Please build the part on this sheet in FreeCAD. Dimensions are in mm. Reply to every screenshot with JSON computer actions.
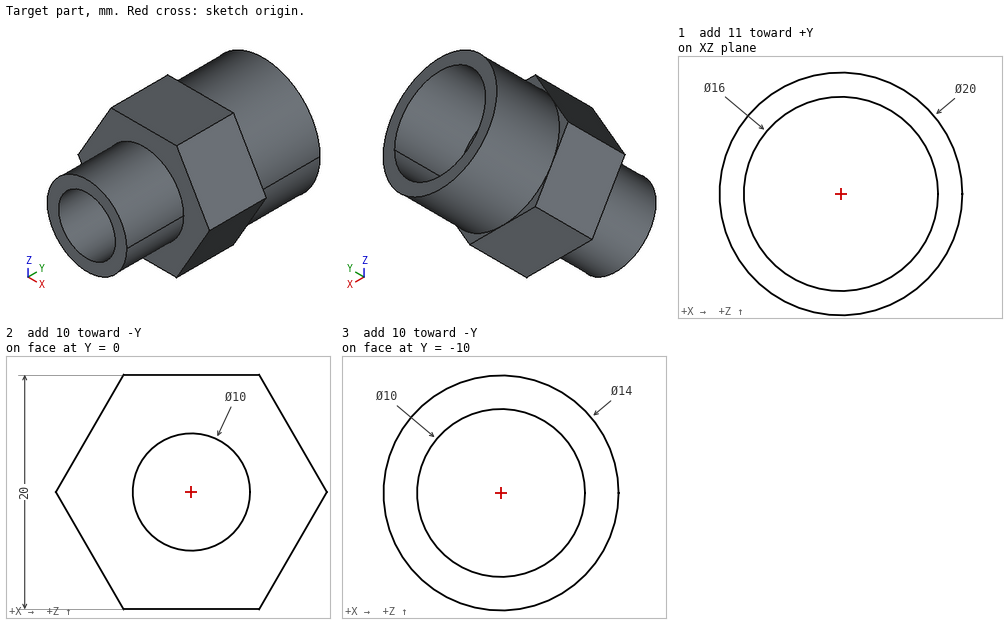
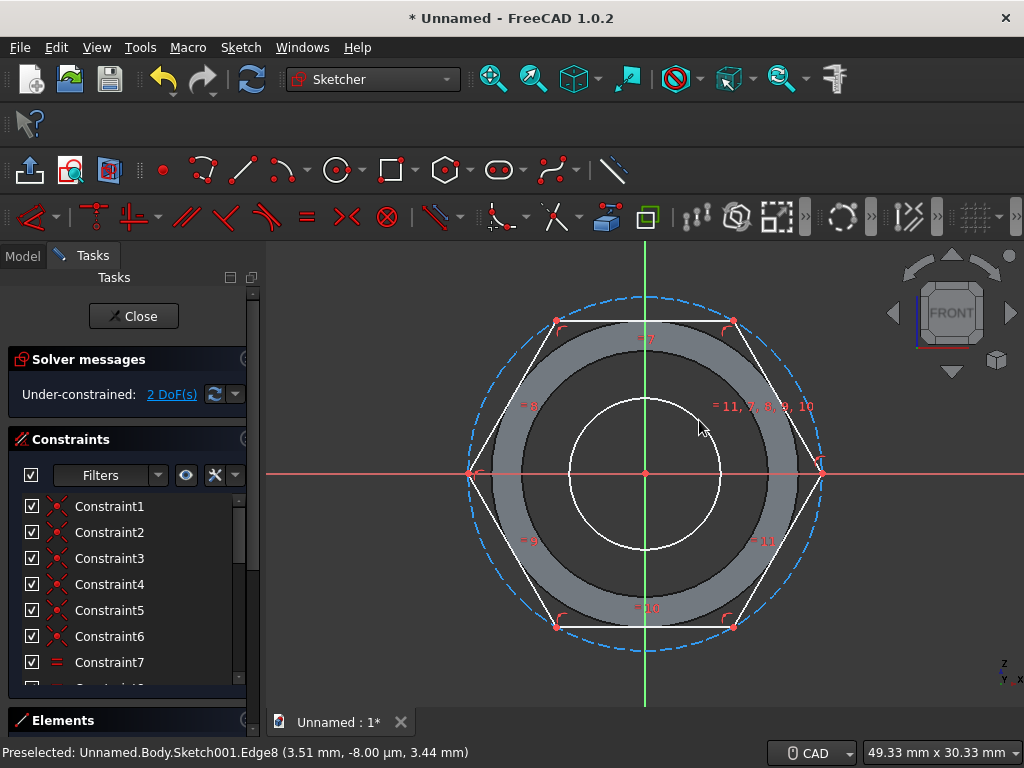
{"action": "left_click", "coordinate": [32, 218]}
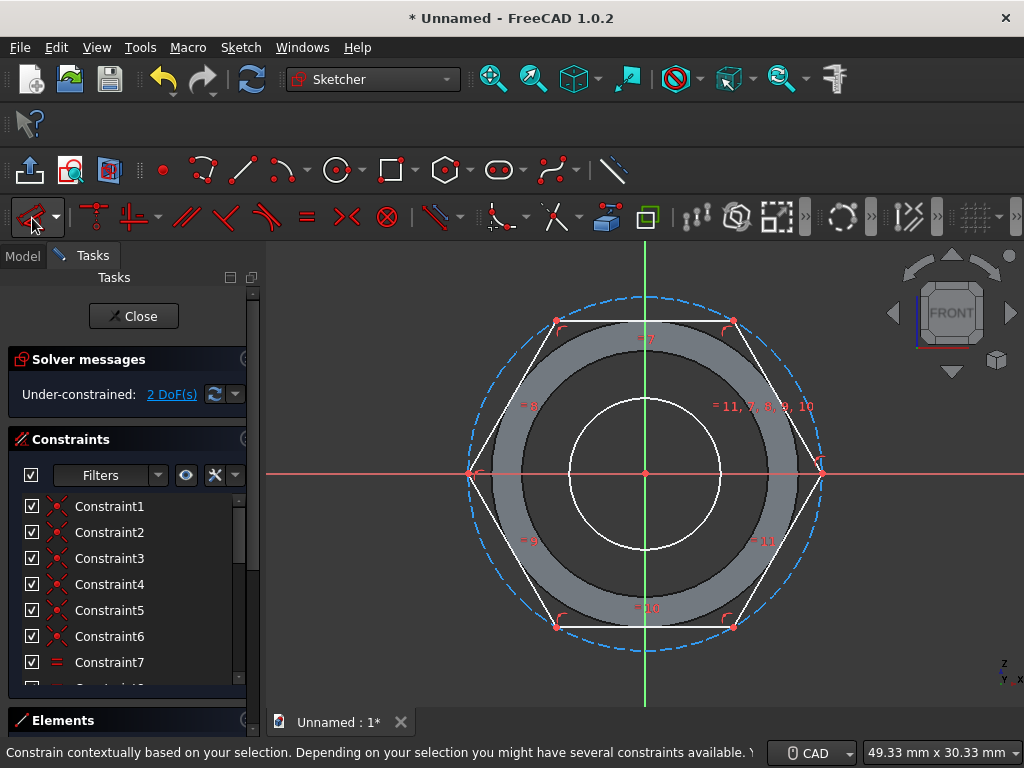
{"action": "left_click", "coordinate": [698, 420]}
{"action": "left_click", "coordinate": [720, 397]}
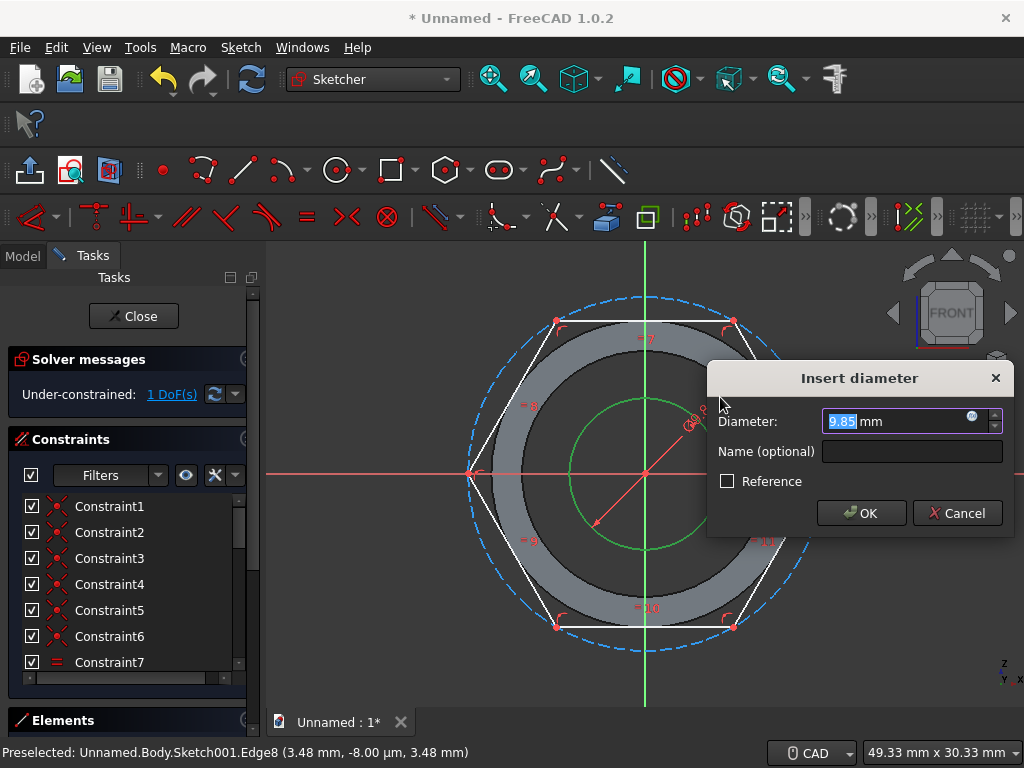
{"action": "type", "text": "10"}
{"action": "key", "text": "Return"}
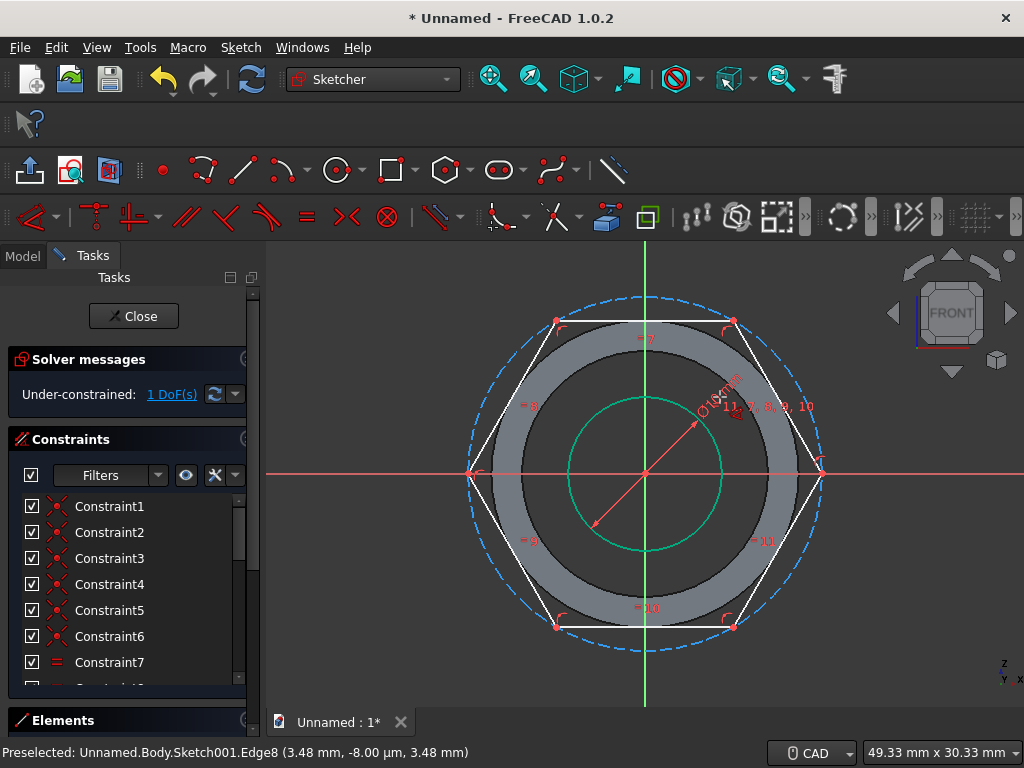
{"action": "left_click", "coordinate": [556, 627]}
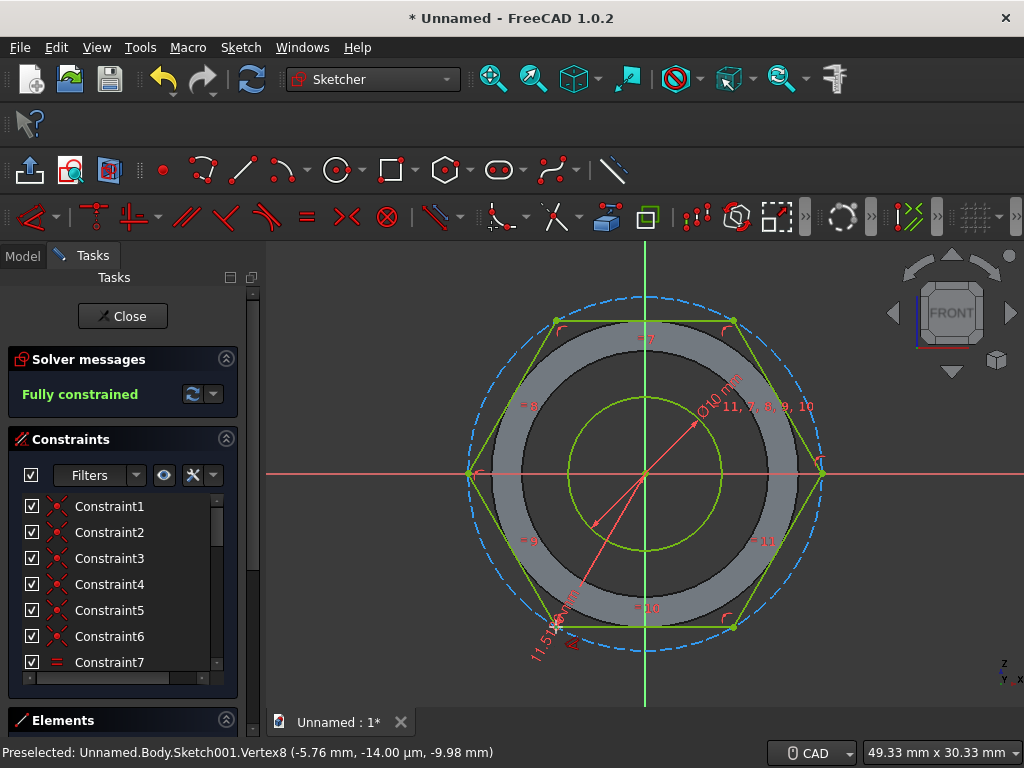
{"action": "left_click", "coordinate": [734, 321]}
{"action": "left_click", "coordinate": [816, 367]}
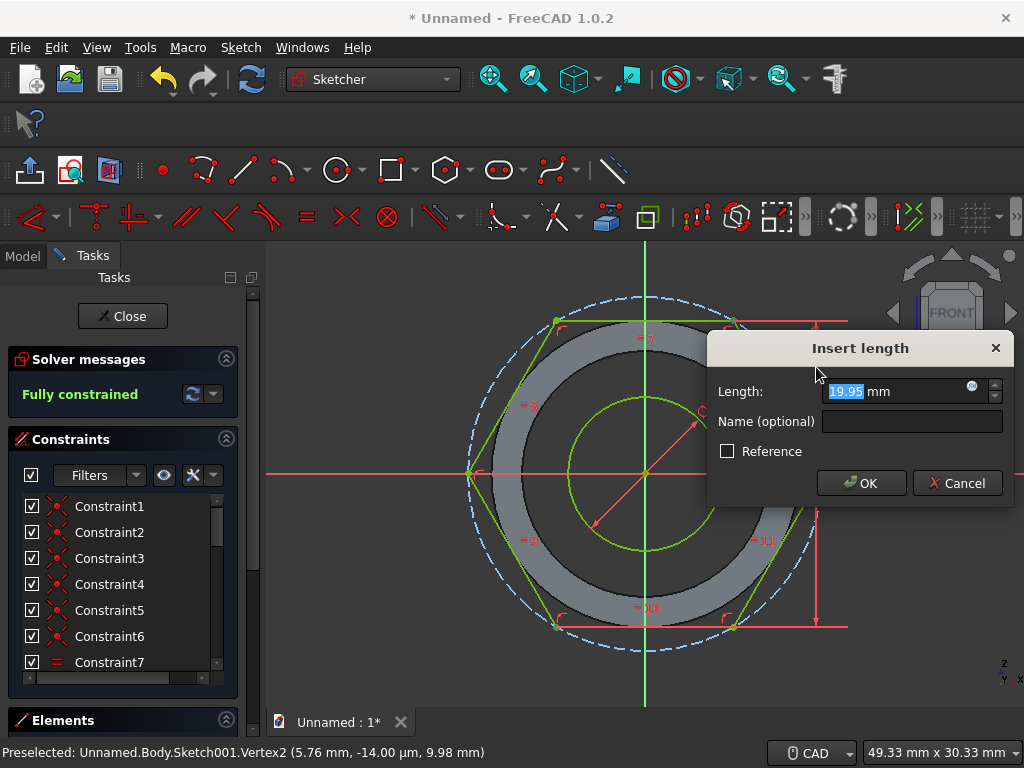
{"action": "type", "text": "20"}
{"action": "key", "text": "Return"}
{"action": "key", "text": "Escape"}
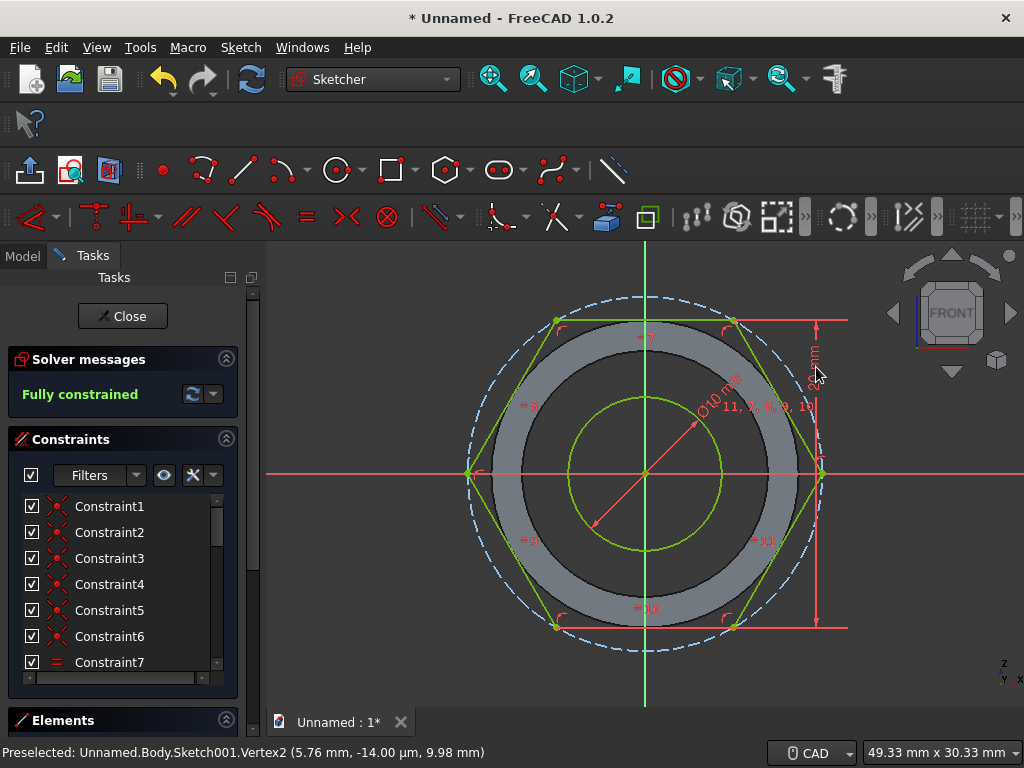
{"action": "left_click", "coordinate": [123, 316]}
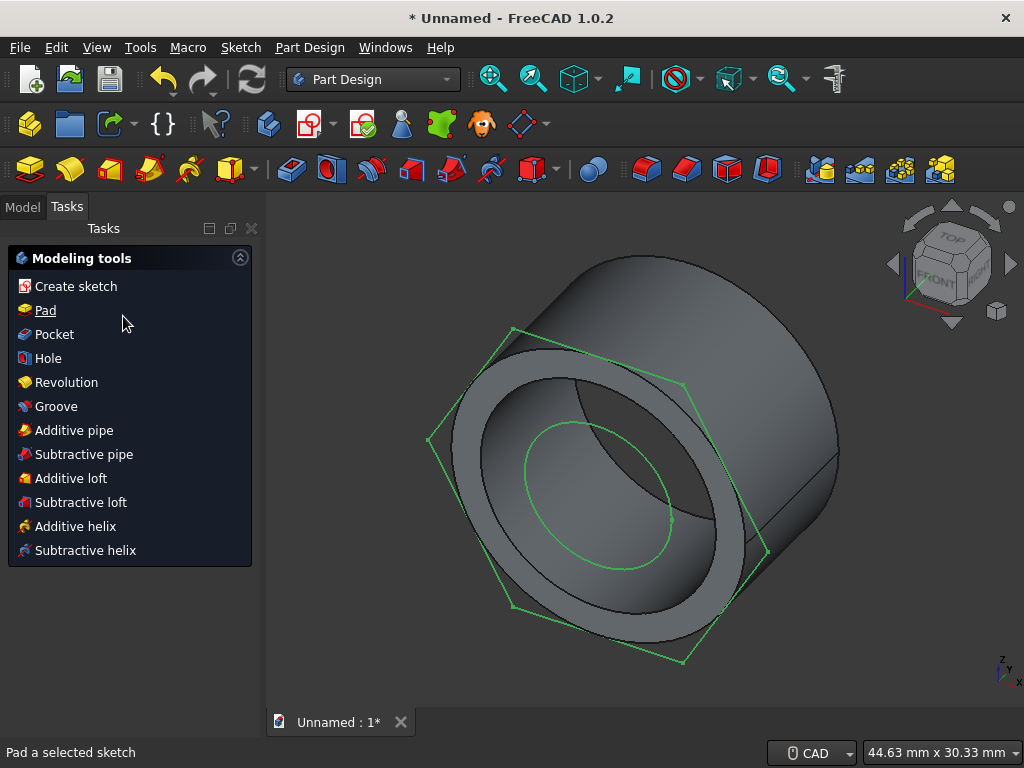
{"action": "left_click", "coordinate": [30, 170]}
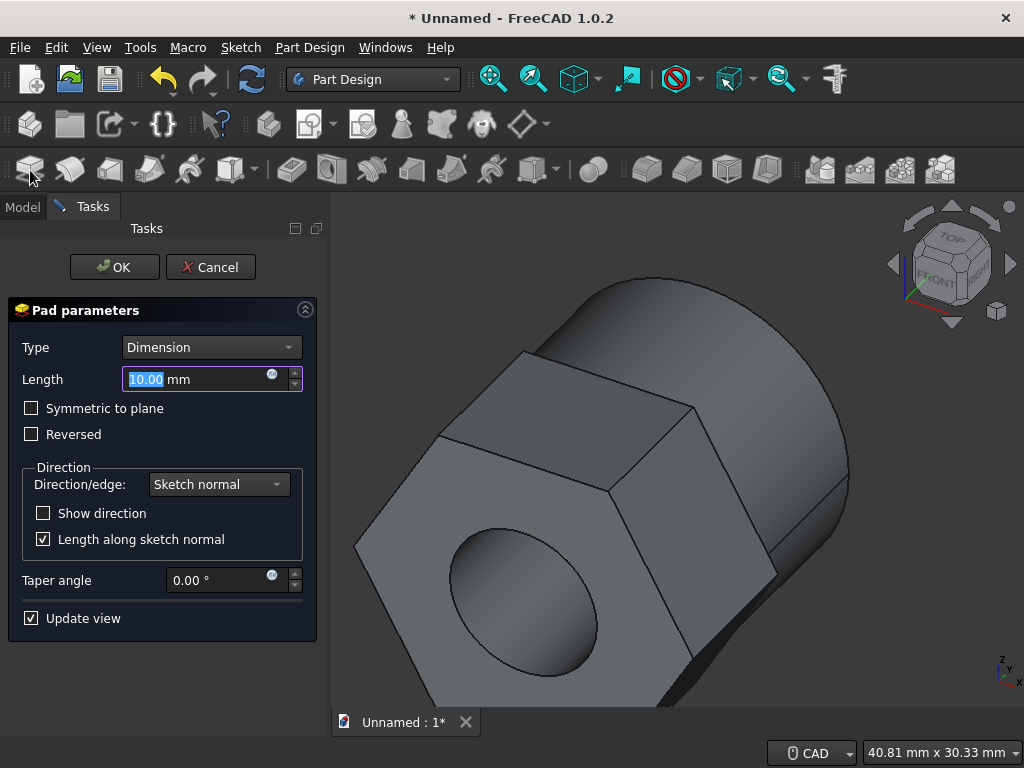
{"action": "type", "text": "10"}
{"action": "key", "text": "Tab"}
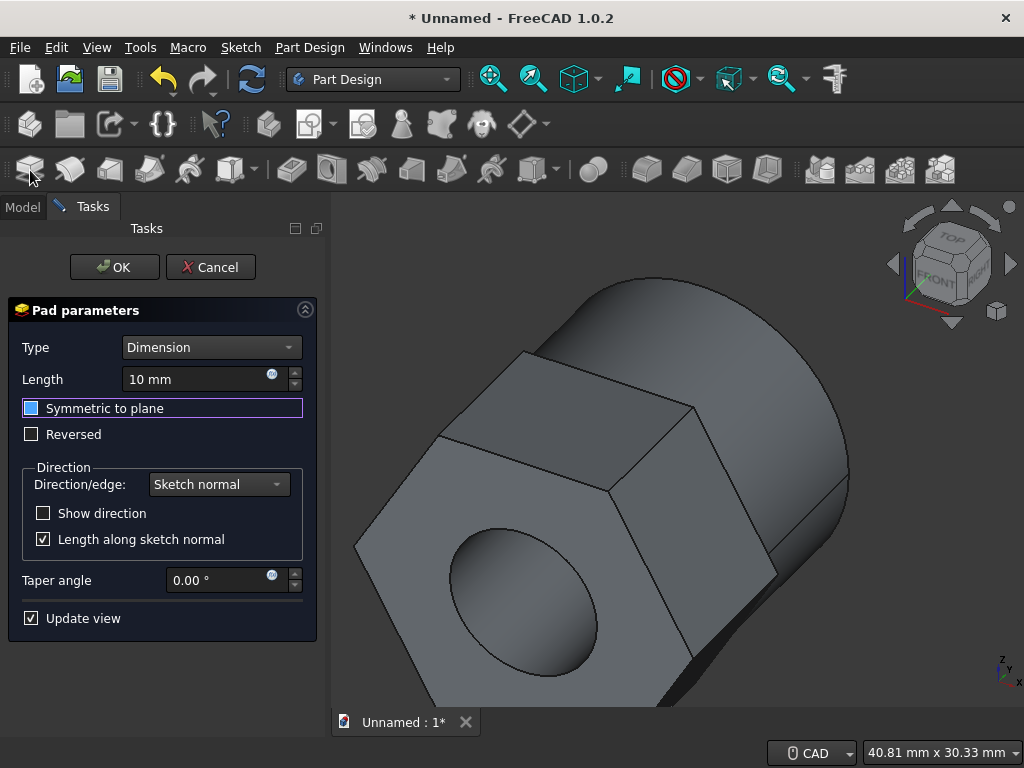
{"action": "left_click", "coordinate": [115, 267]}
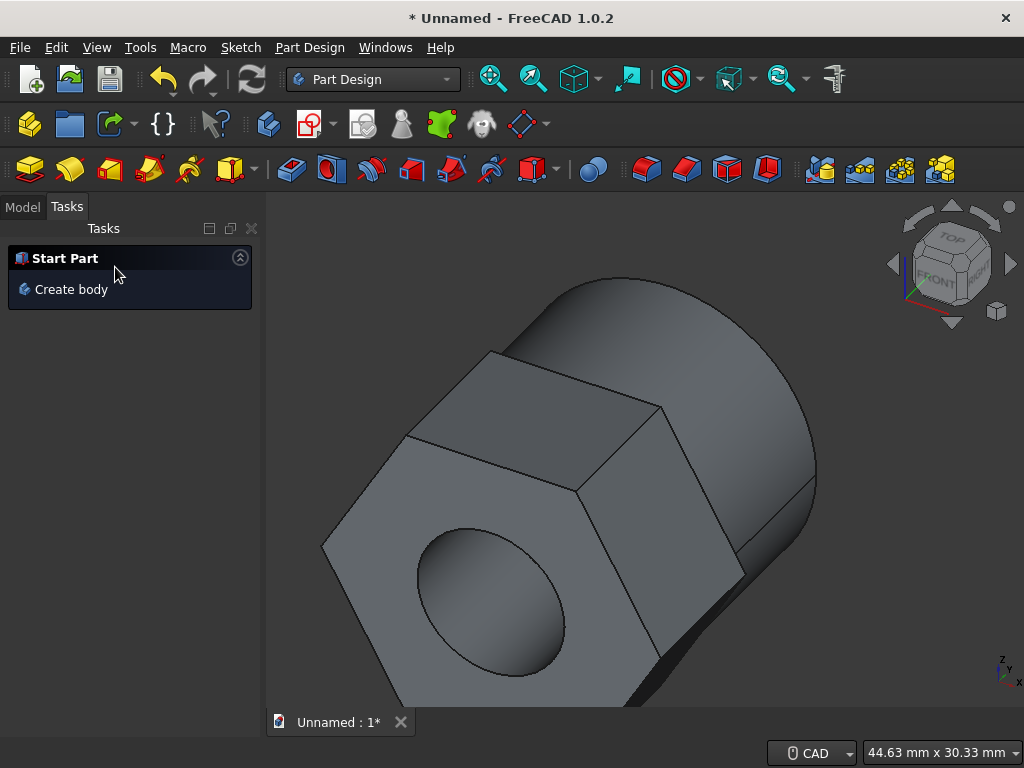
{"action": "left_click", "coordinate": [494, 80]}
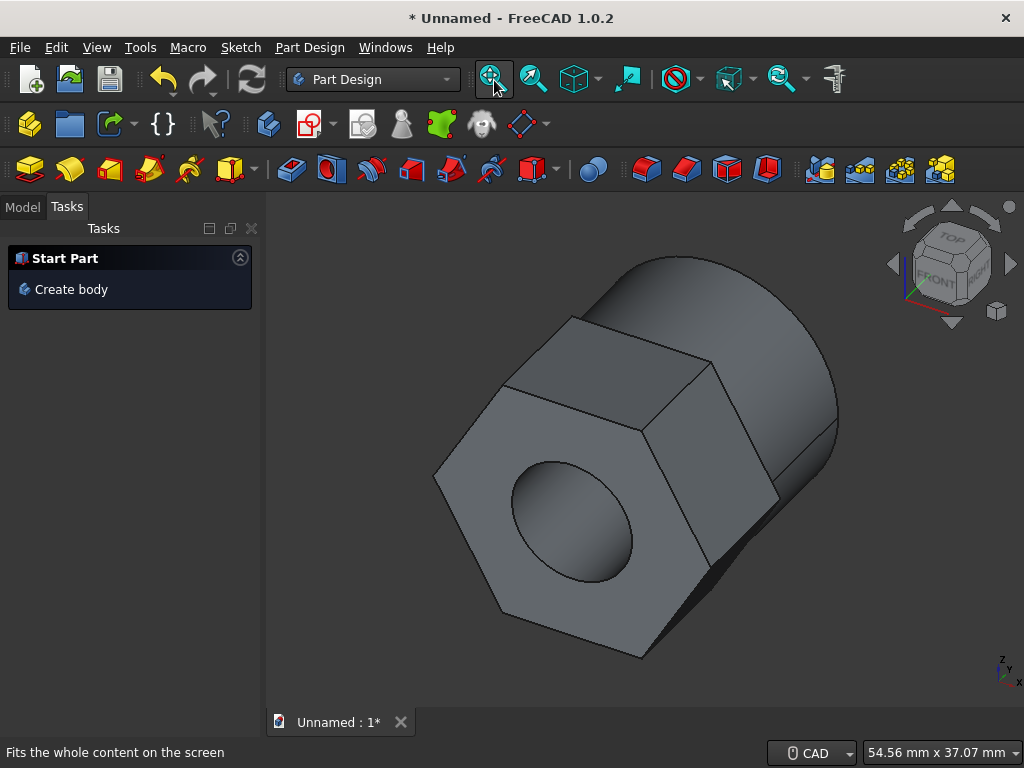
{"action": "left_click", "coordinate": [493, 527]}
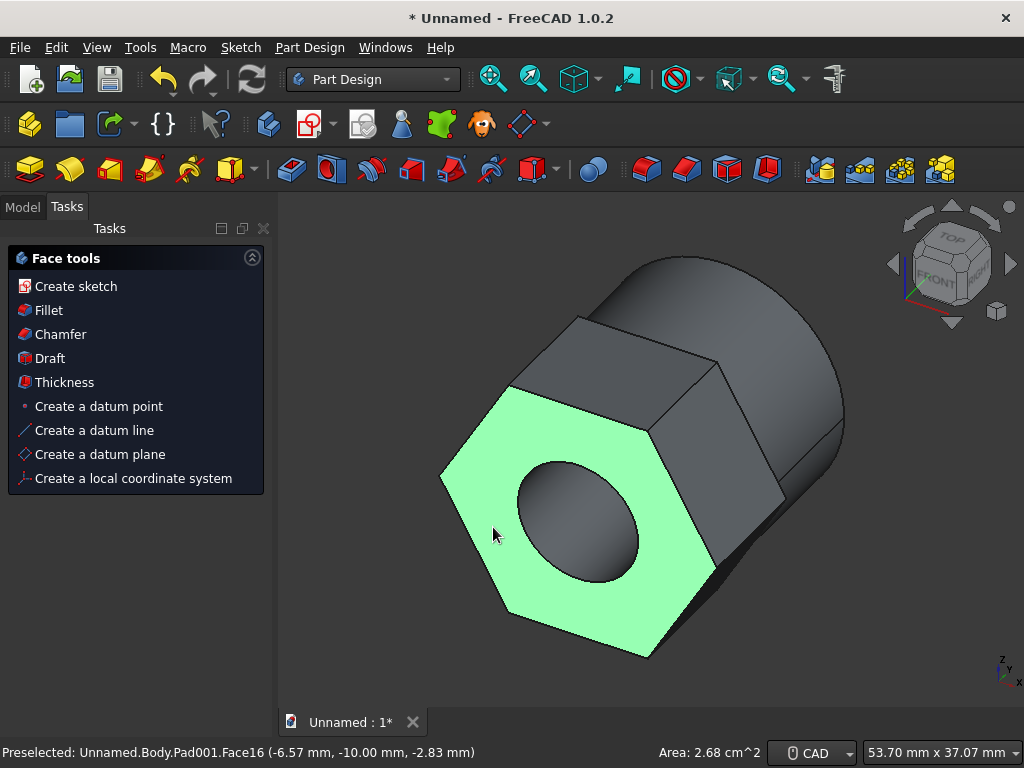
{"action": "left_click", "coordinate": [310, 124]}